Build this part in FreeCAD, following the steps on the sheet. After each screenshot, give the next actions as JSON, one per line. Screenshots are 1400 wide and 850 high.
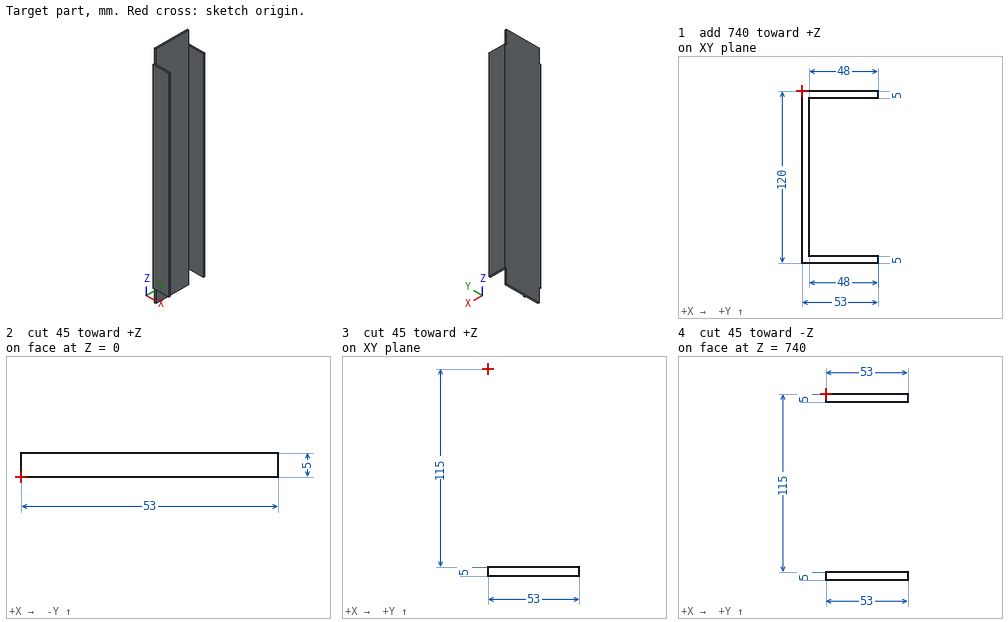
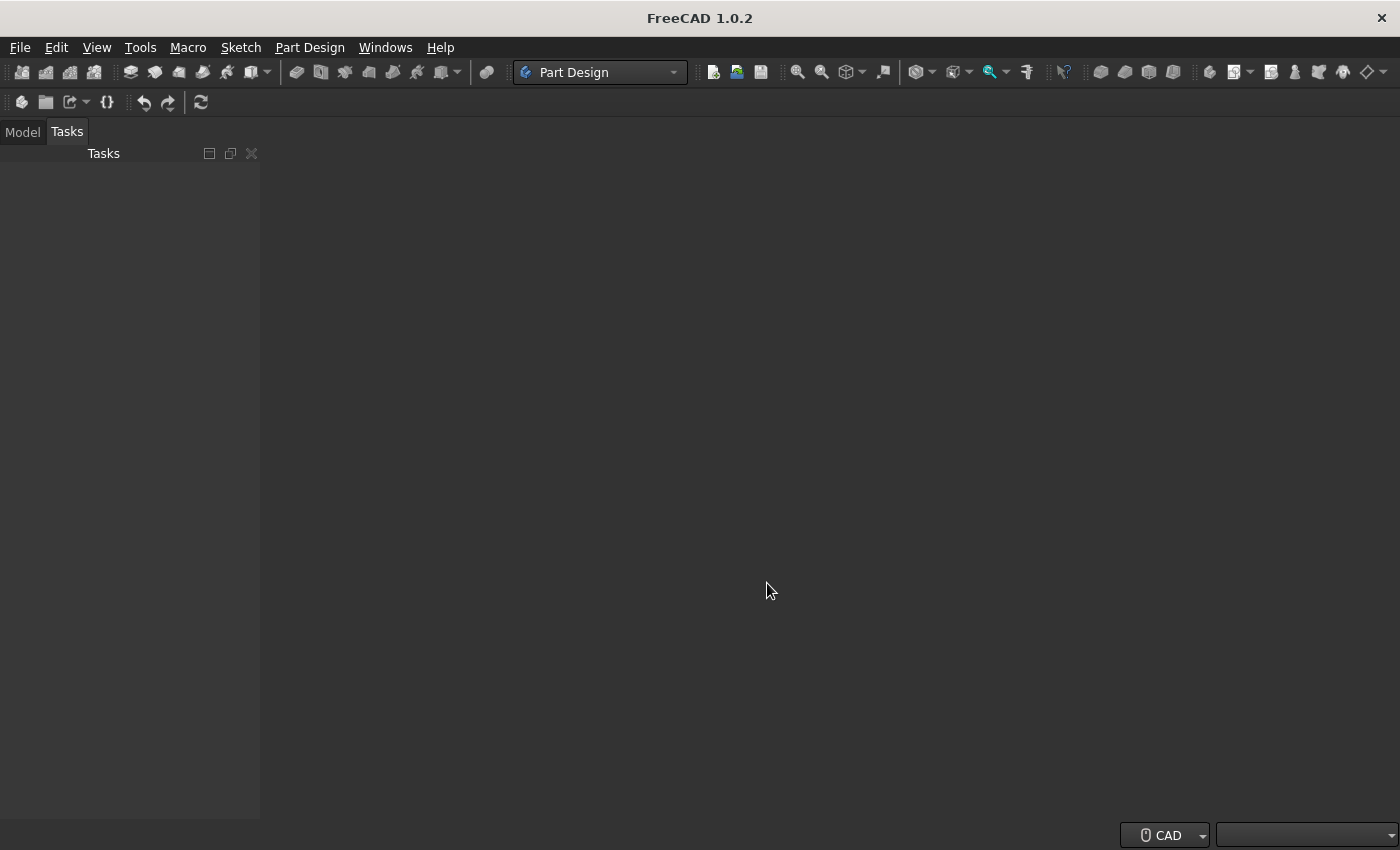
{"action": "left_click", "coordinate": [714, 72]}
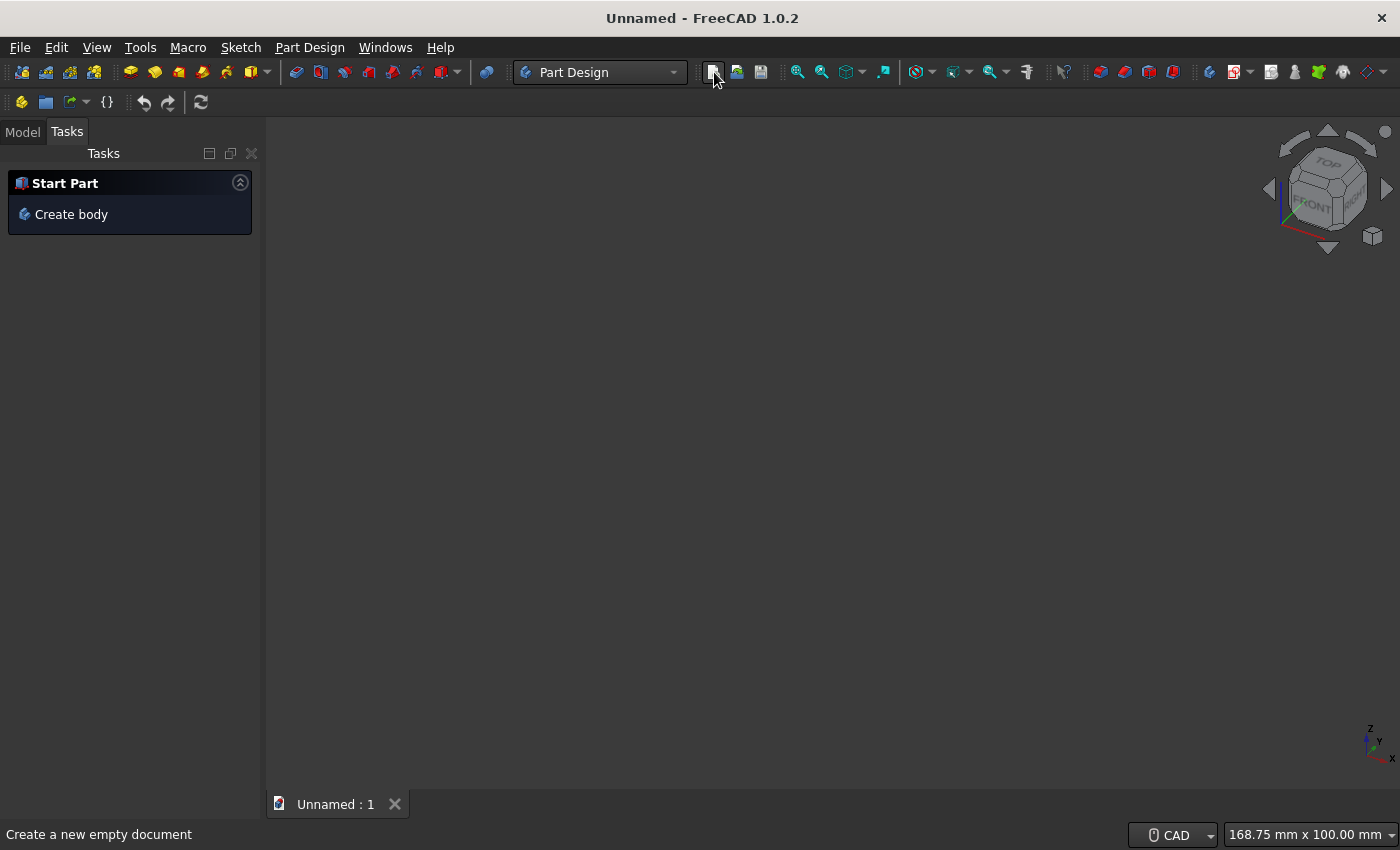
{"action": "left_click", "coordinate": [1234, 72]}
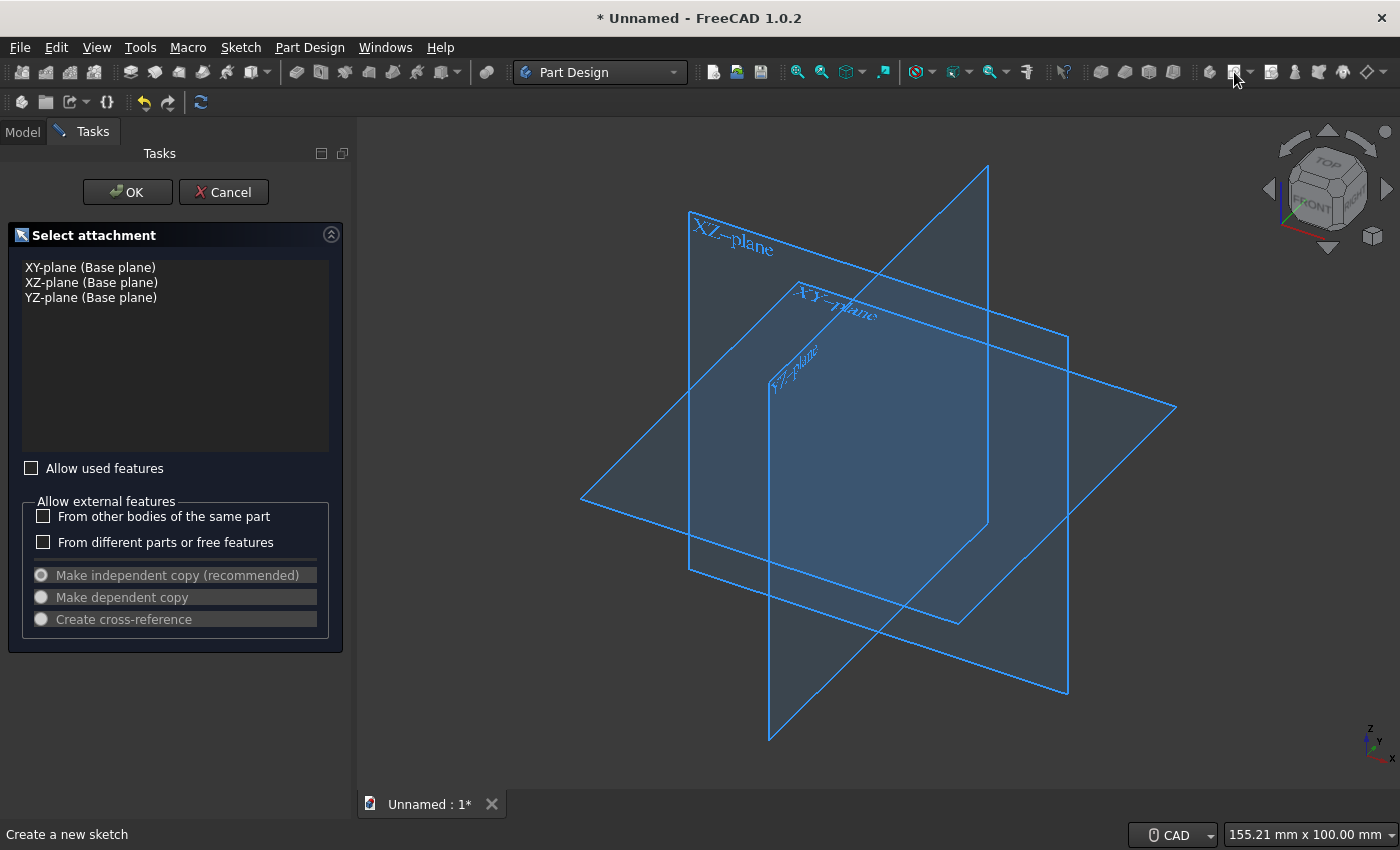
{"action": "left_click", "coordinate": [82, 268]}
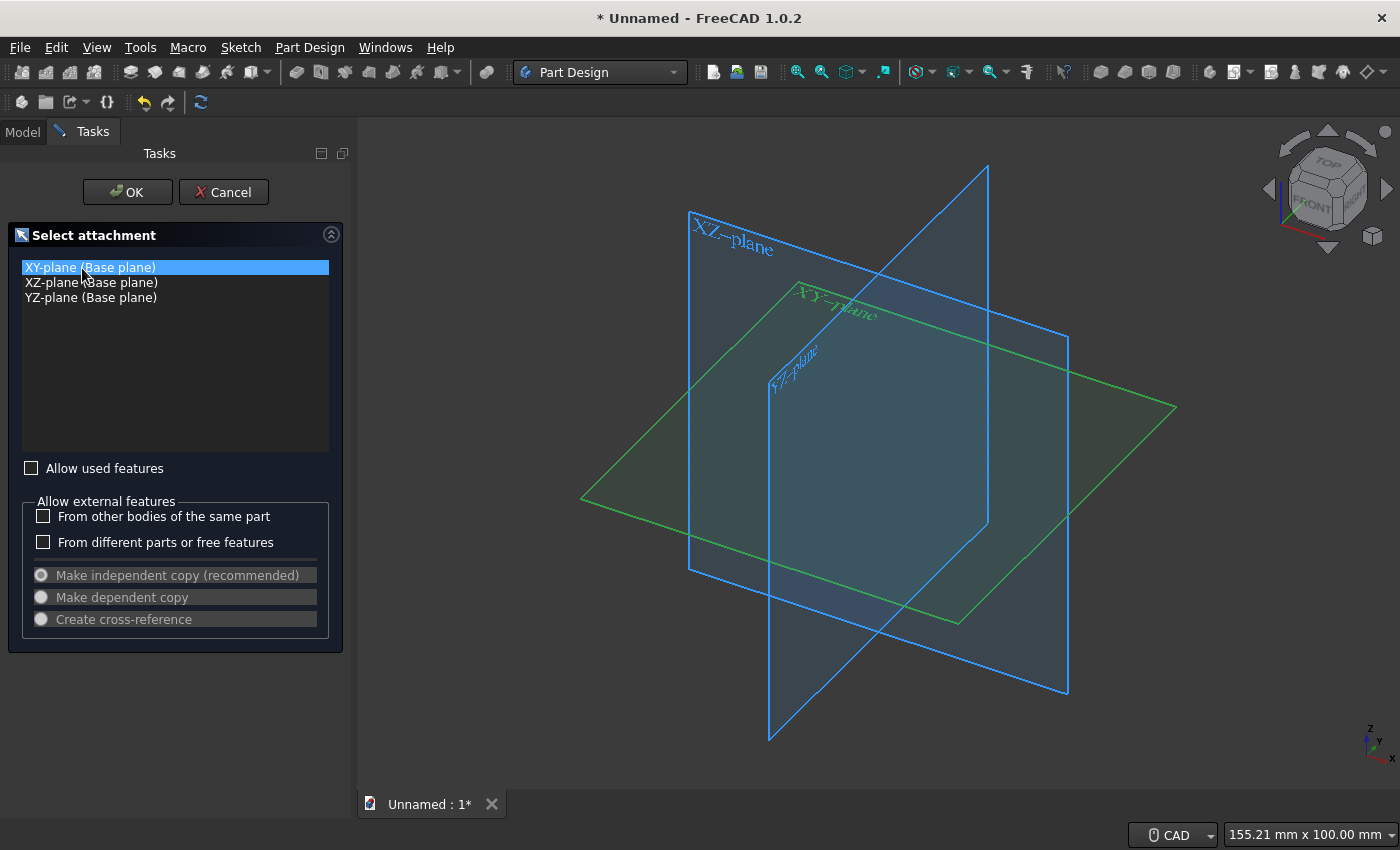
{"action": "left_click", "coordinate": [128, 192]}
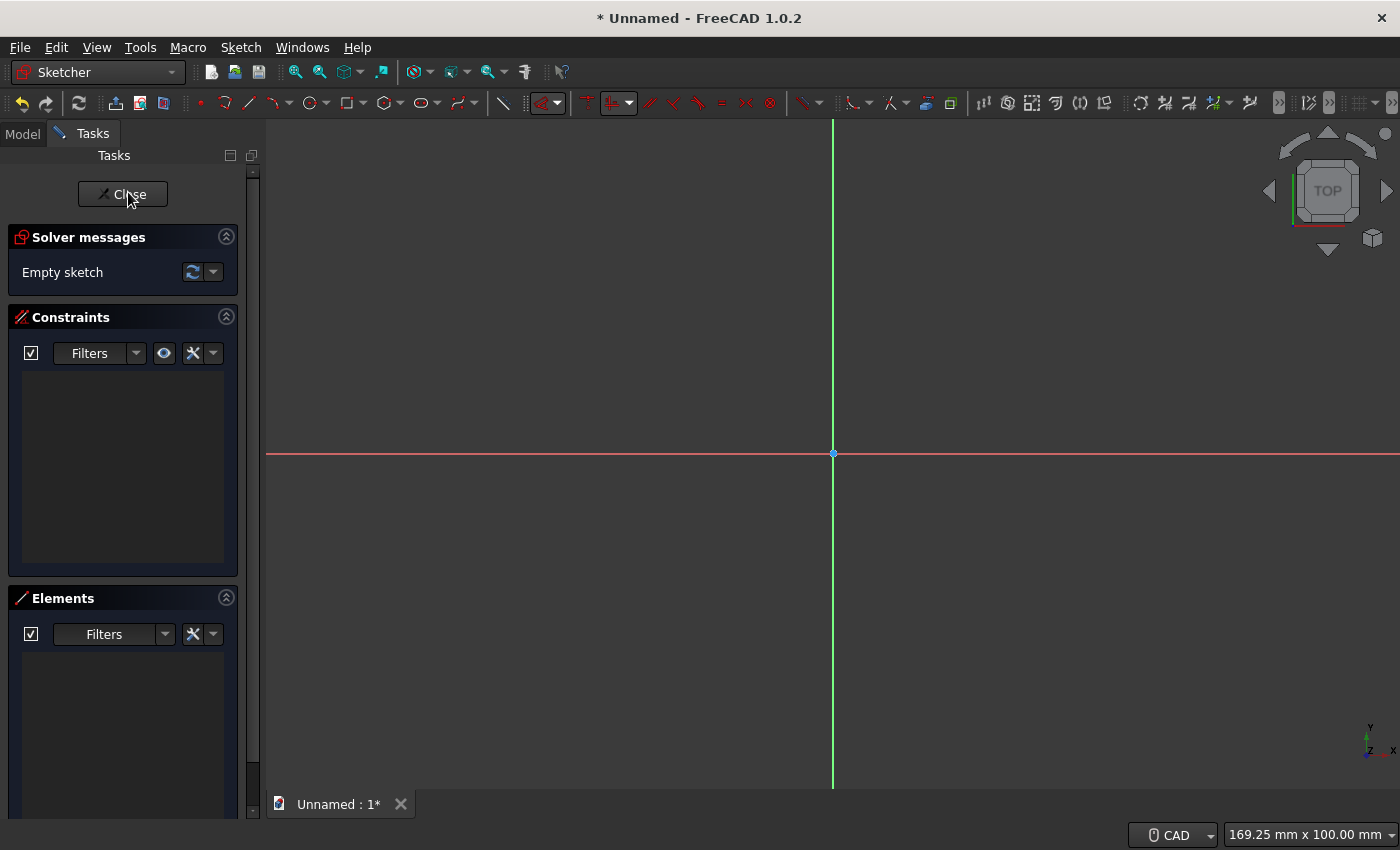
{"action": "scroll", "coordinate": [564, 147], "scroll_direction": "down", "scroll_amount": 4}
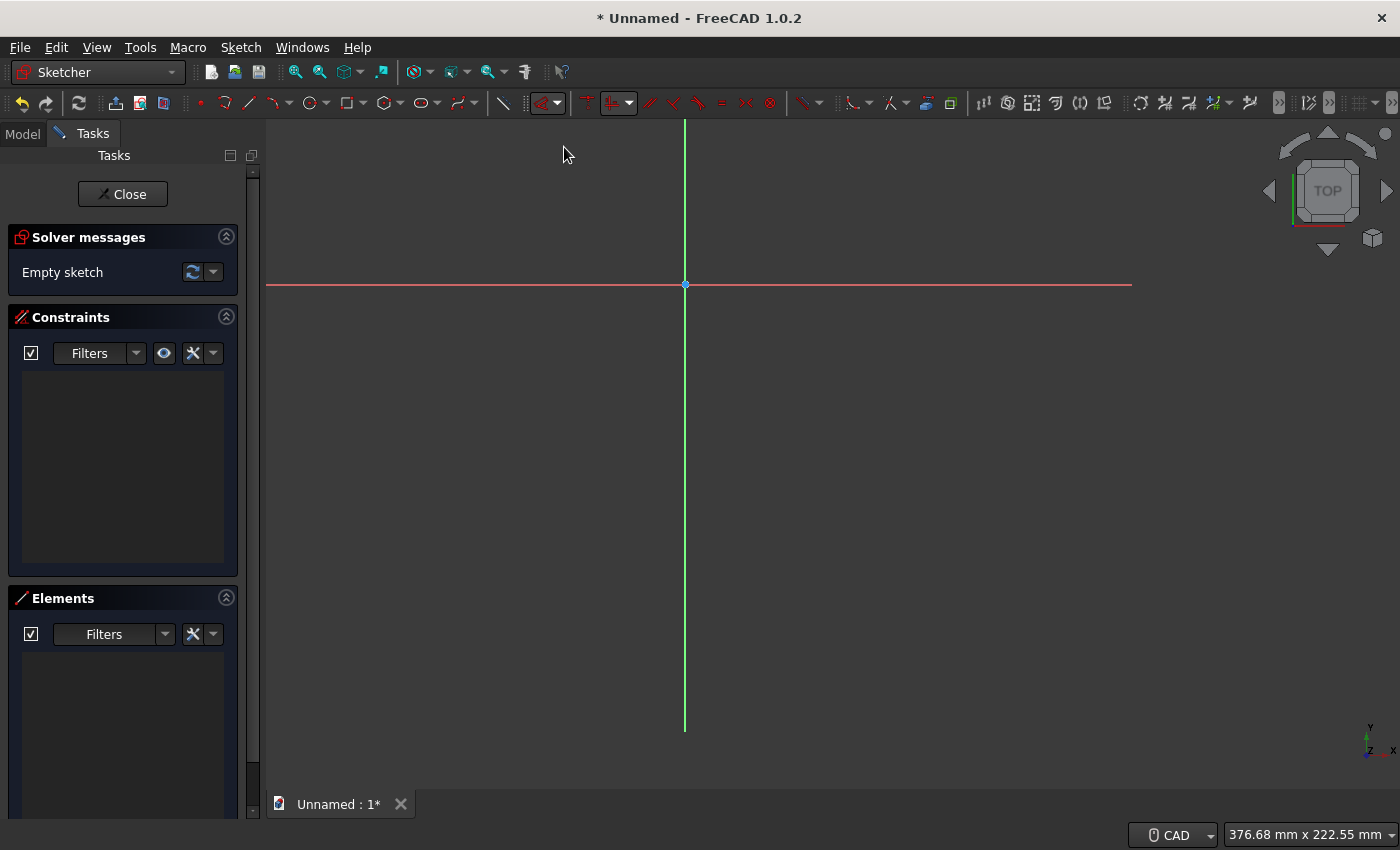
{"action": "left_click", "coordinate": [226, 104]}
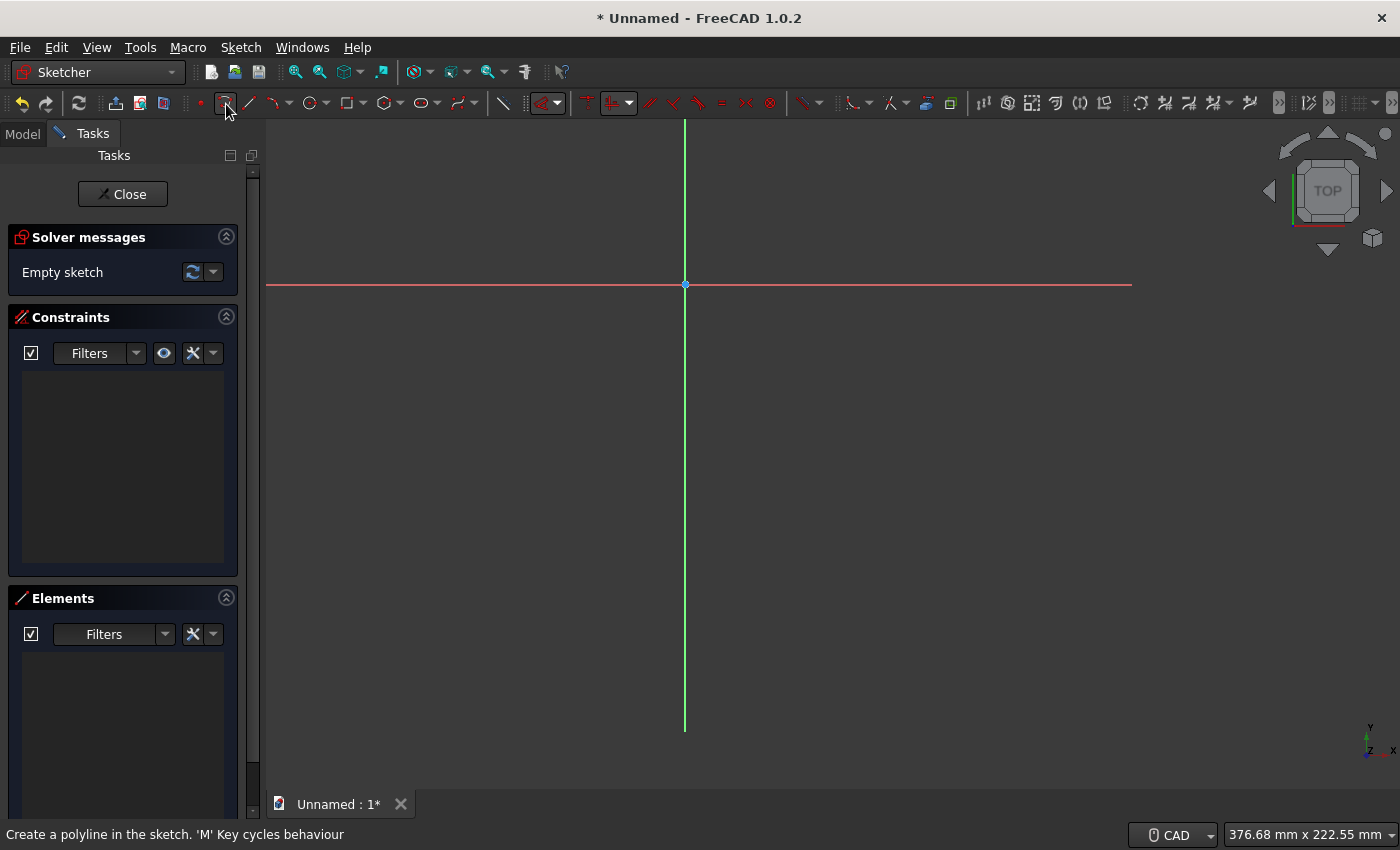
{"action": "left_click", "coordinate": [685, 285]}
{"action": "left_click", "coordinate": [694, 646]}
{"action": "left_click", "coordinate": [845, 646]}
{"action": "left_click", "coordinate": [845, 631]}
{"action": "left_click", "coordinate": [700, 631]}
{"action": "left_click", "coordinate": [700, 300]}
{"action": "left_click", "coordinate": [845, 300]}
{"action": "left_click", "coordinate": [845, 294]}
{"action": "left_click", "coordinate": [685, 285]}
{"action": "key", "text": "Escape"}
{"action": "key", "text": "Escape"}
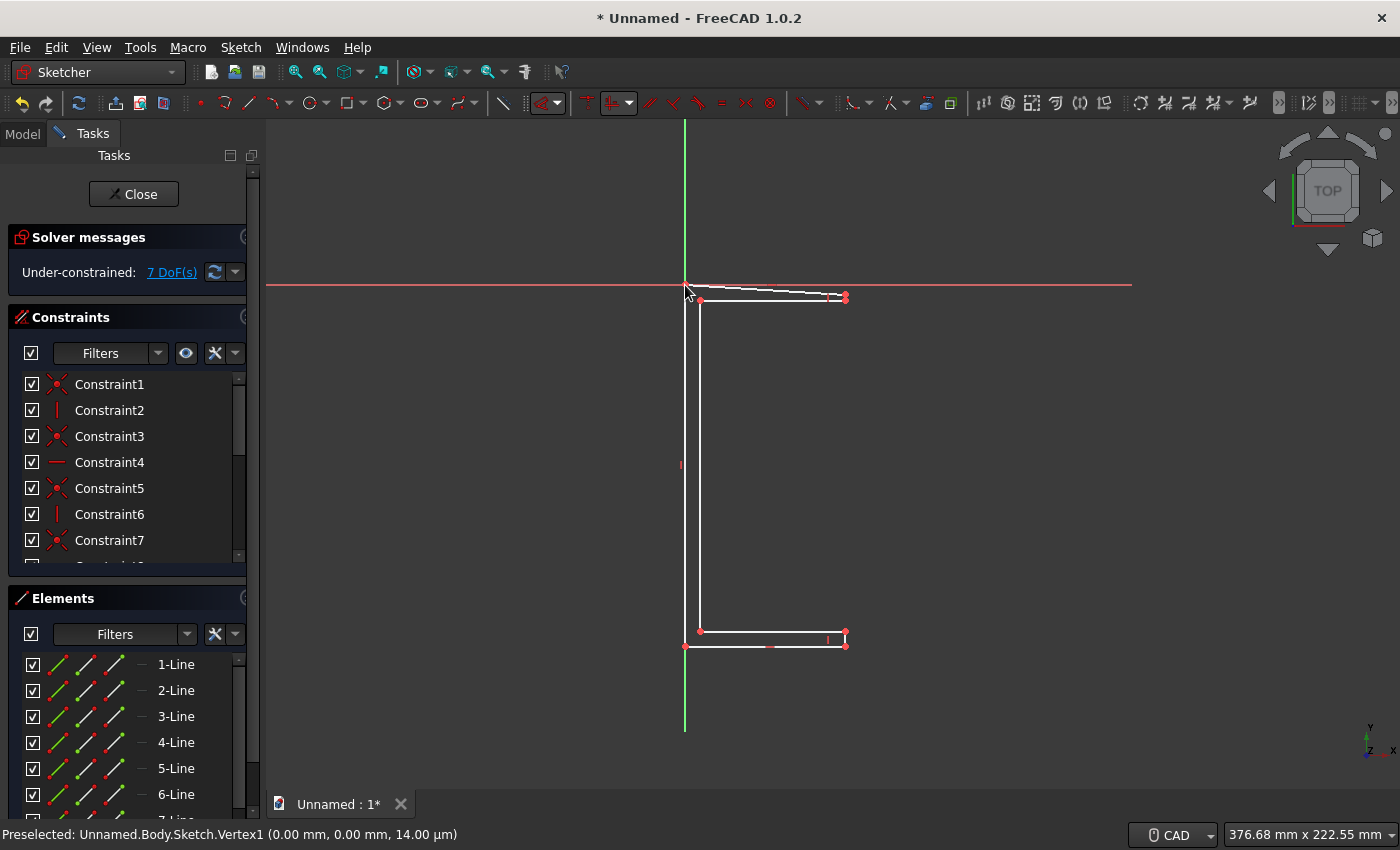
{"action": "left_click", "coordinate": [733, 288]}